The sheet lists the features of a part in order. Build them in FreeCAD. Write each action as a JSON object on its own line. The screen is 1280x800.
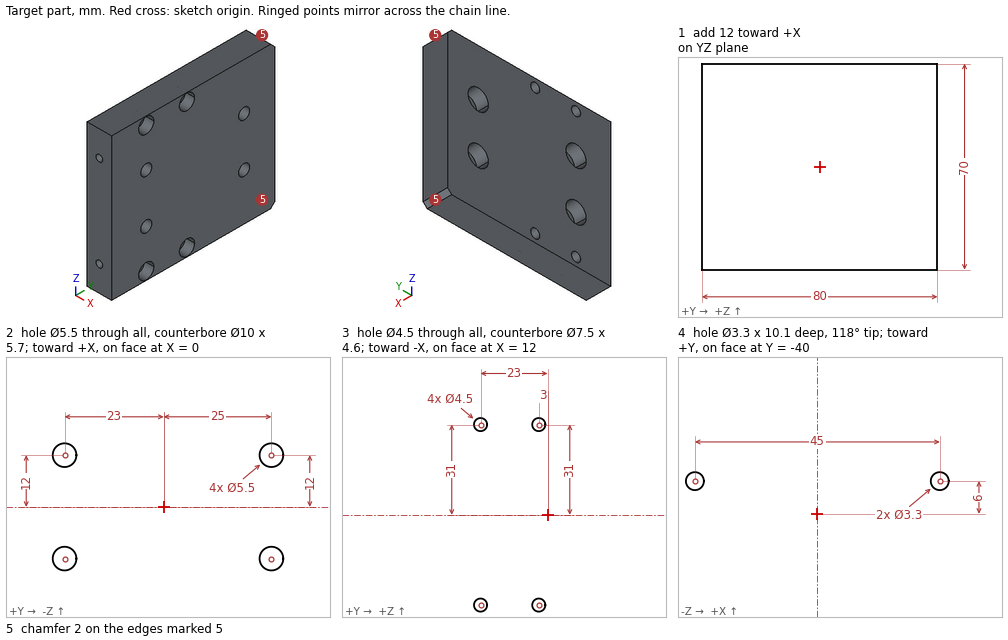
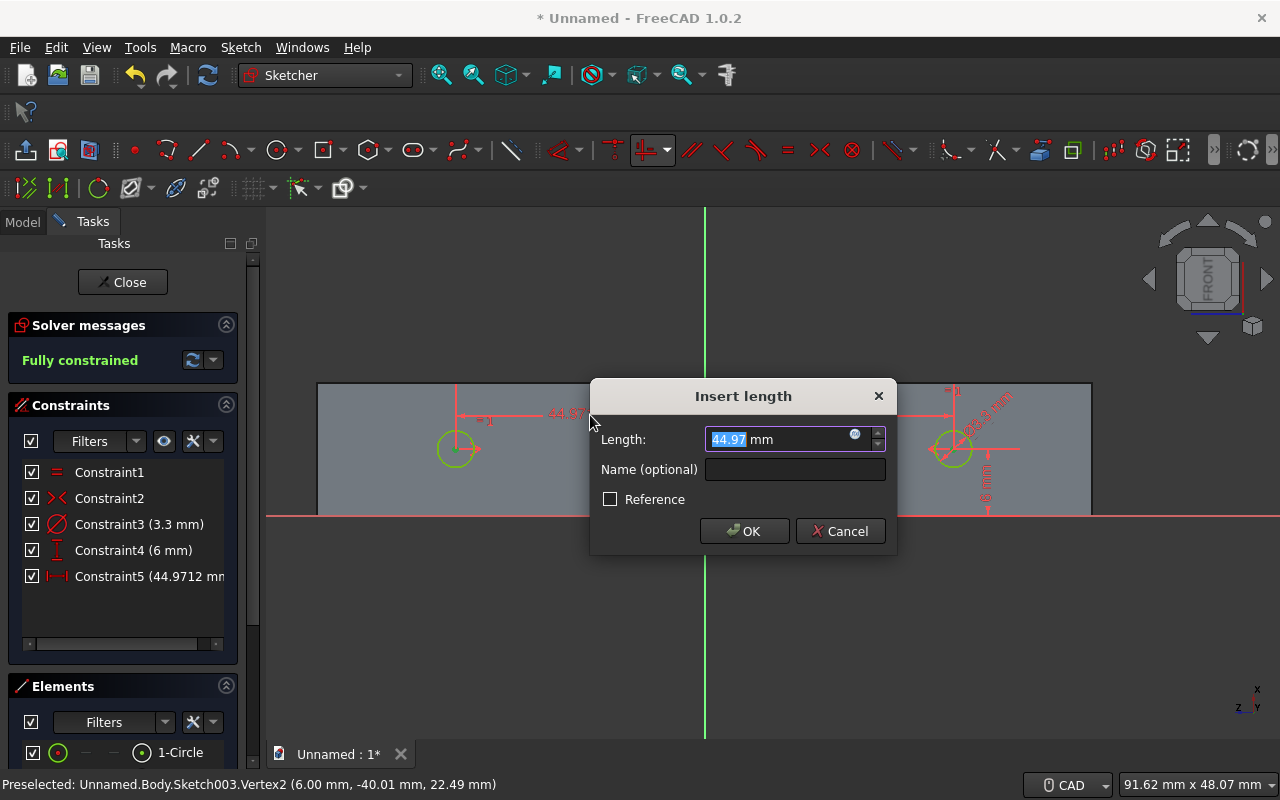
{"action": "type", "text": "45"}
{"action": "key", "text": "Return"}
{"action": "key", "text": "Escape"}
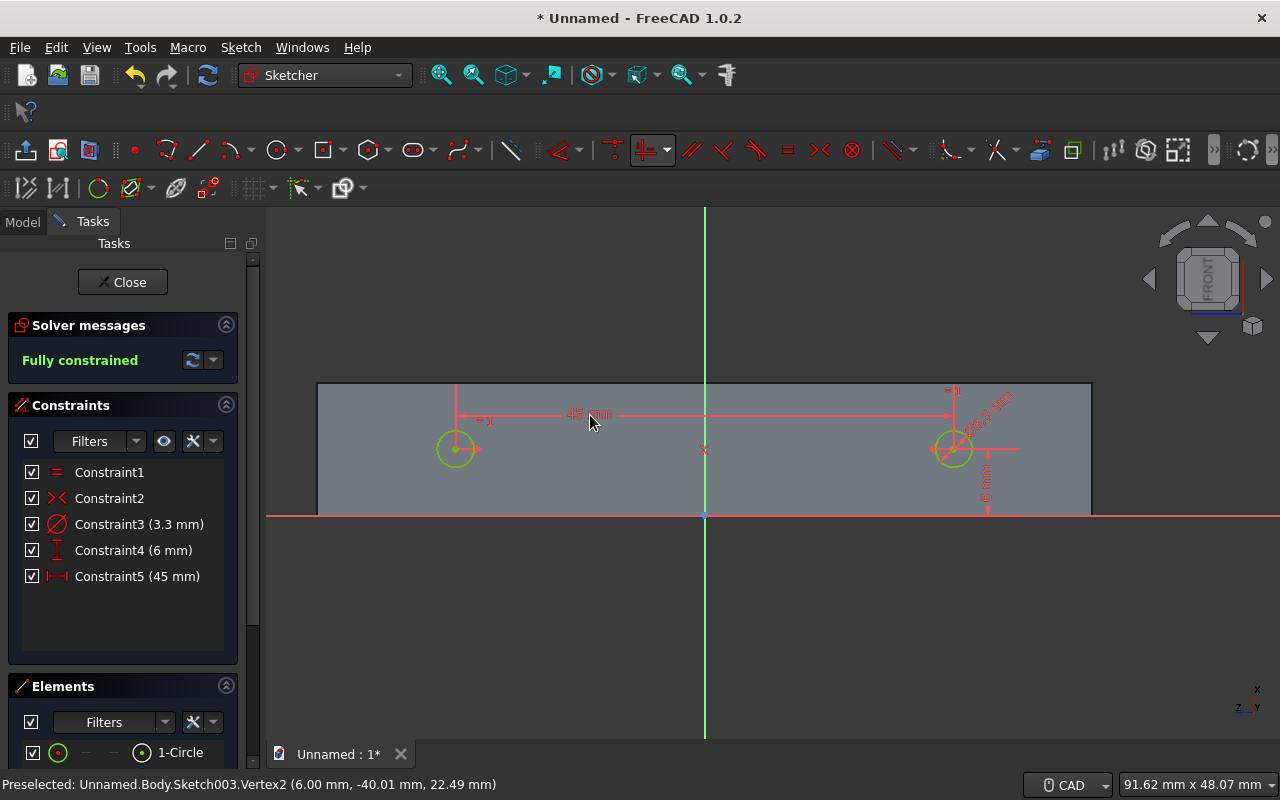
{"action": "left_click", "coordinate": [123, 282]}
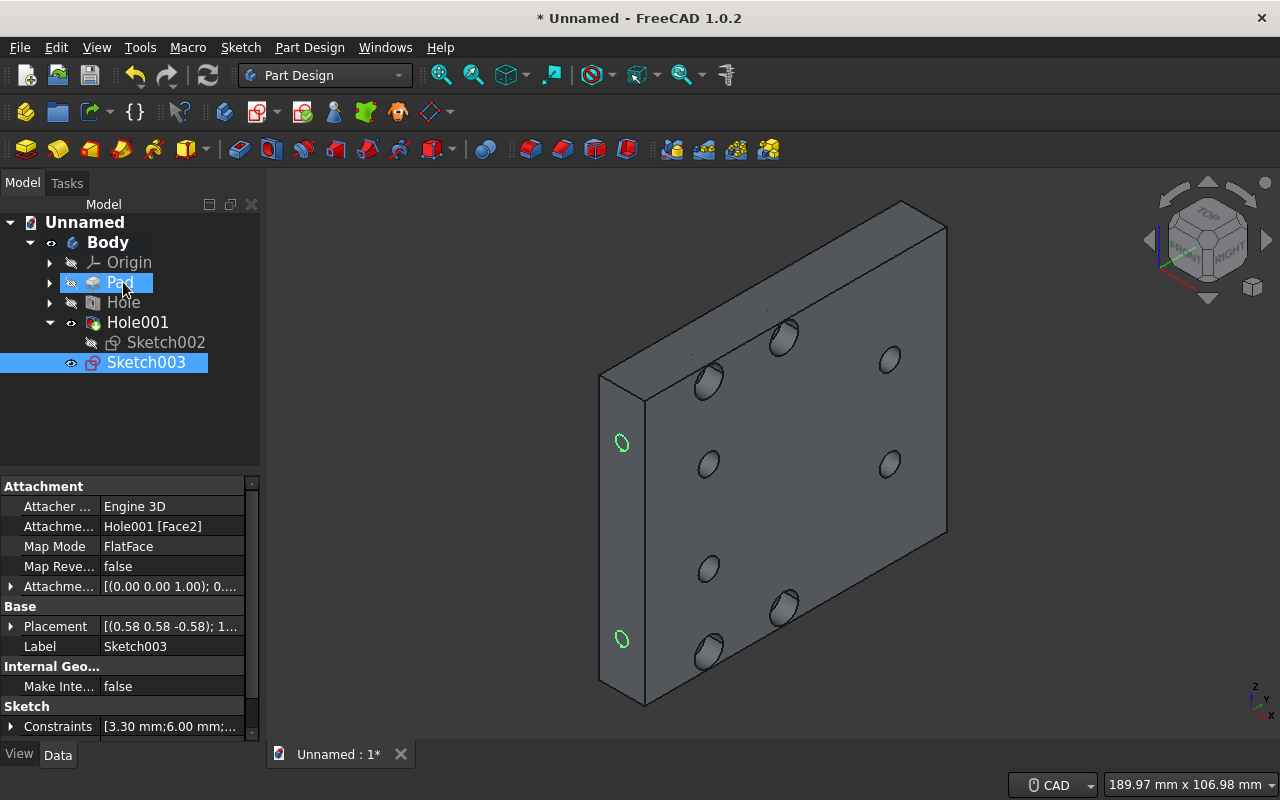
{"action": "left_click", "coordinate": [272, 150]}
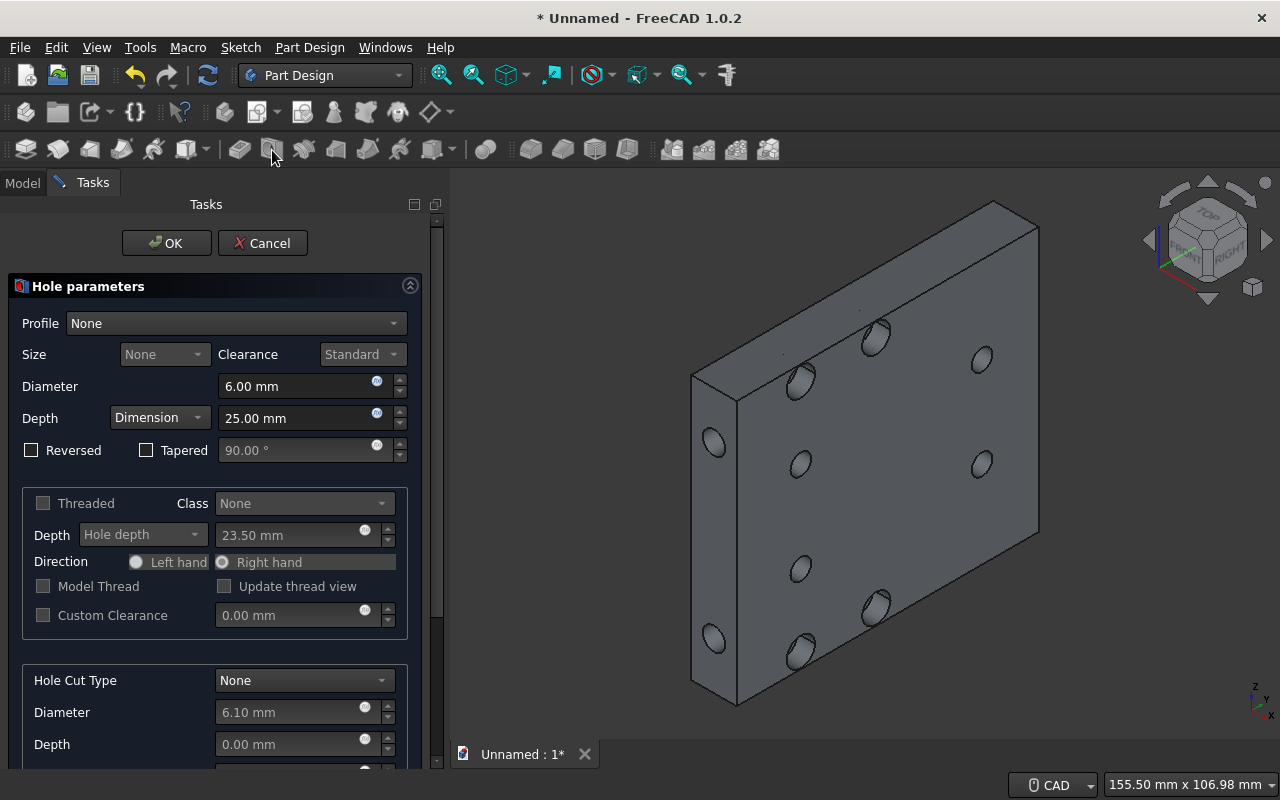
{"action": "triple_click", "coordinate": [305, 386]}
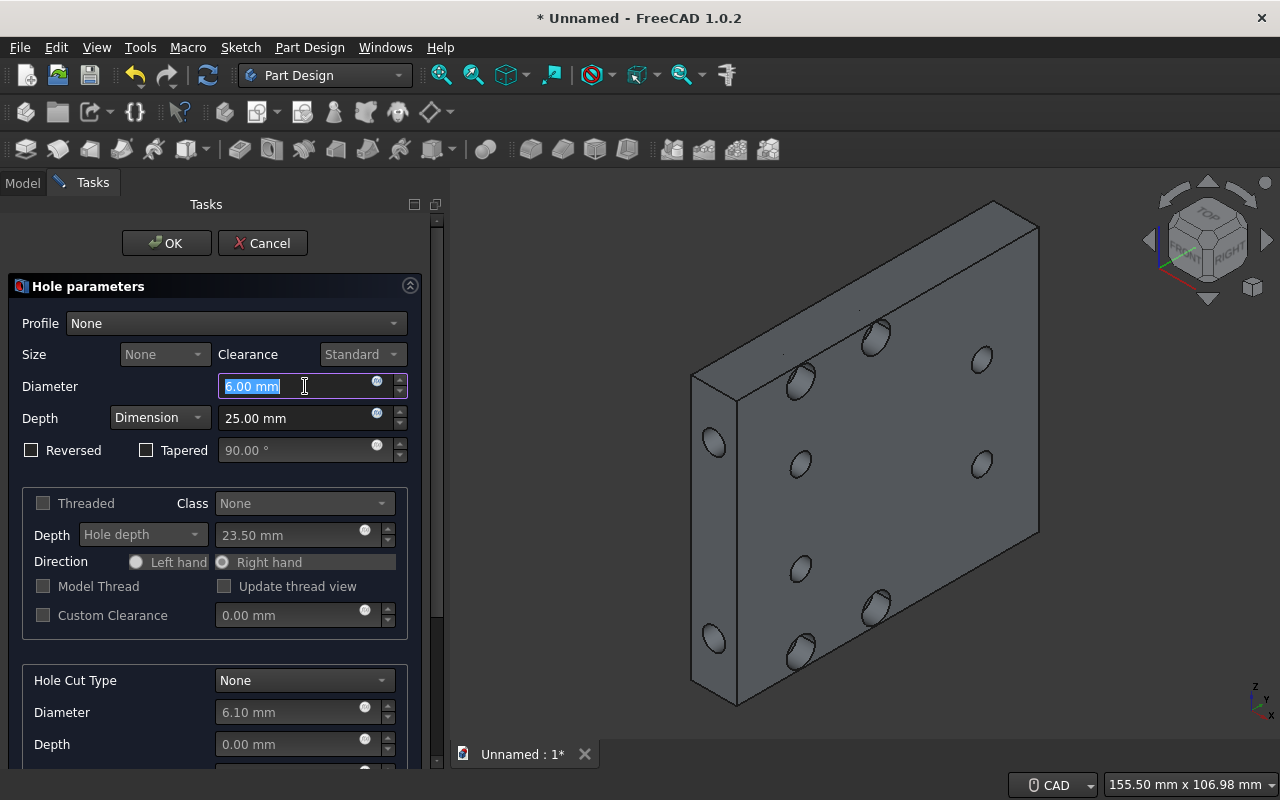
{"action": "type", "text": "3.3"}
{"action": "key", "text": "Tab"}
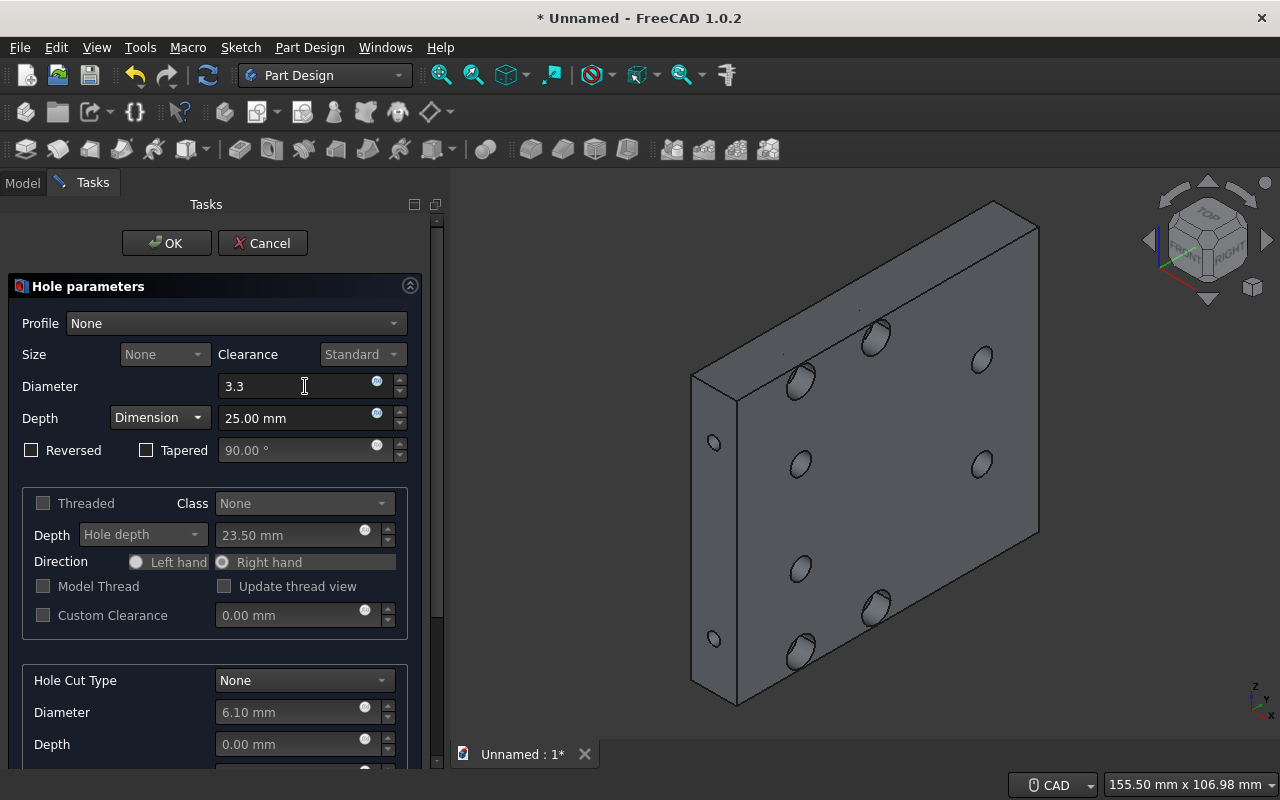
{"action": "triple_click", "coordinate": [305, 418]}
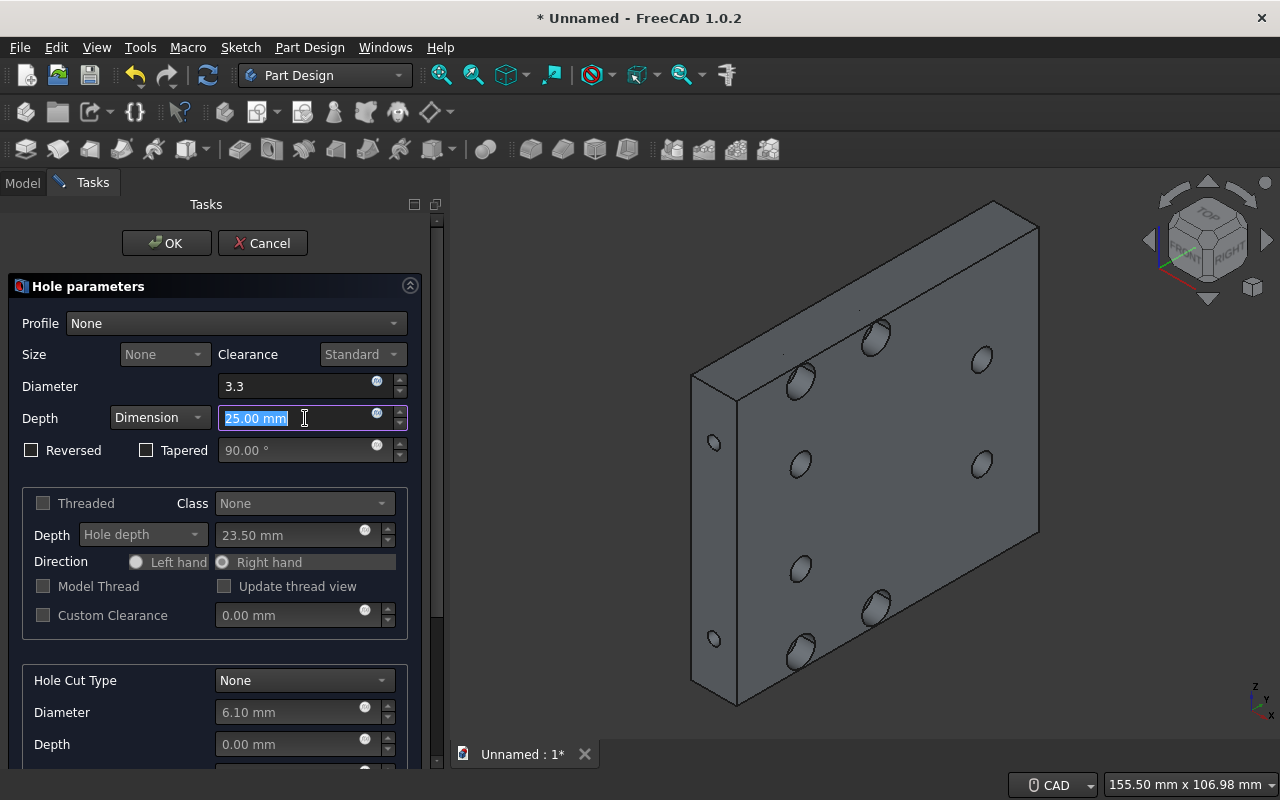
{"action": "type", "text": "10.1"}
{"action": "key", "text": "Tab"}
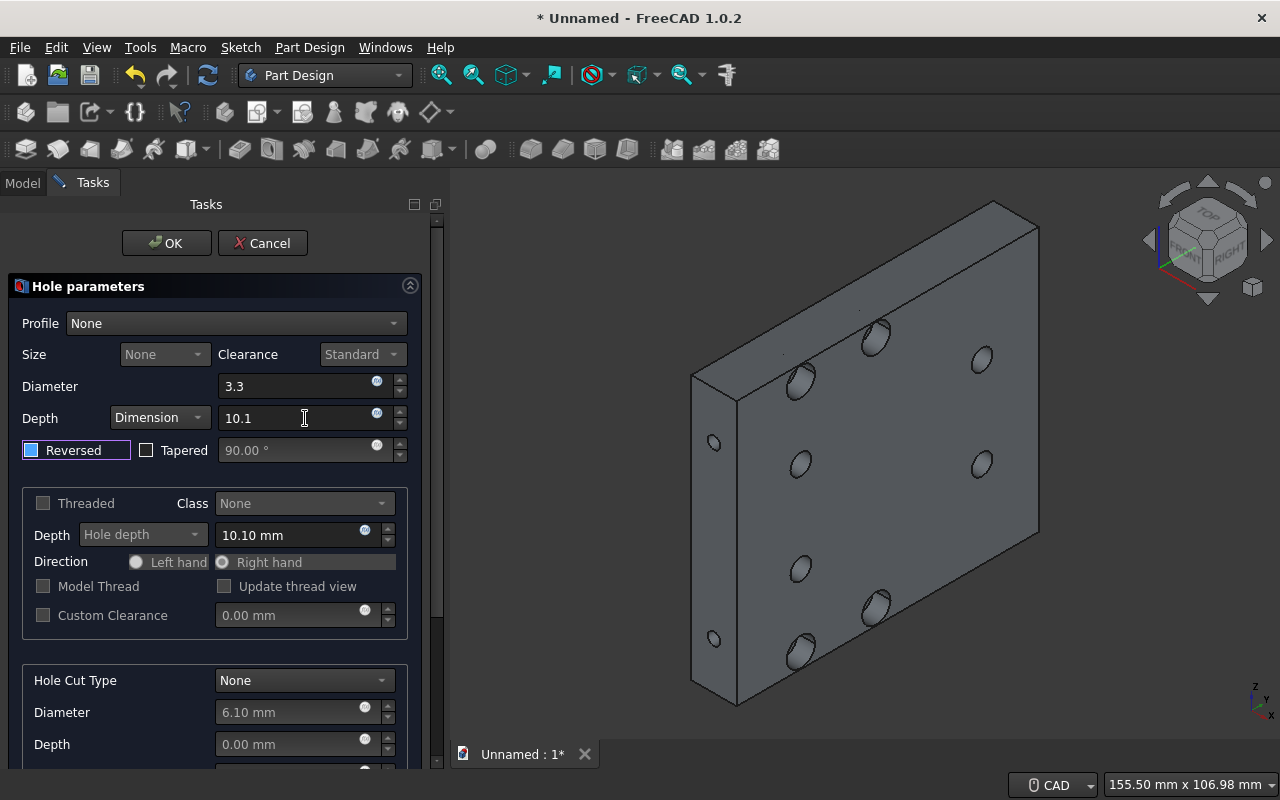
{"action": "left_click", "coordinate": [167, 243]}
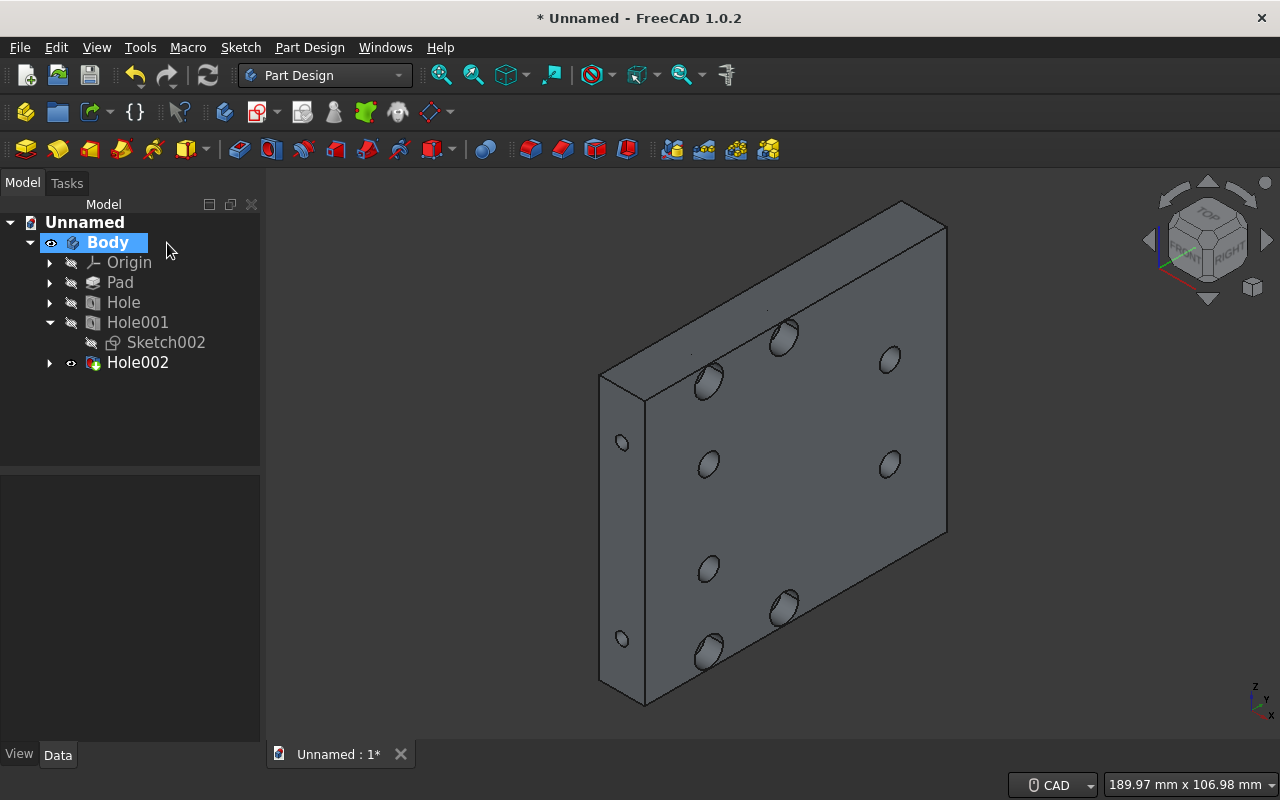
{"action": "key", "text": "2"}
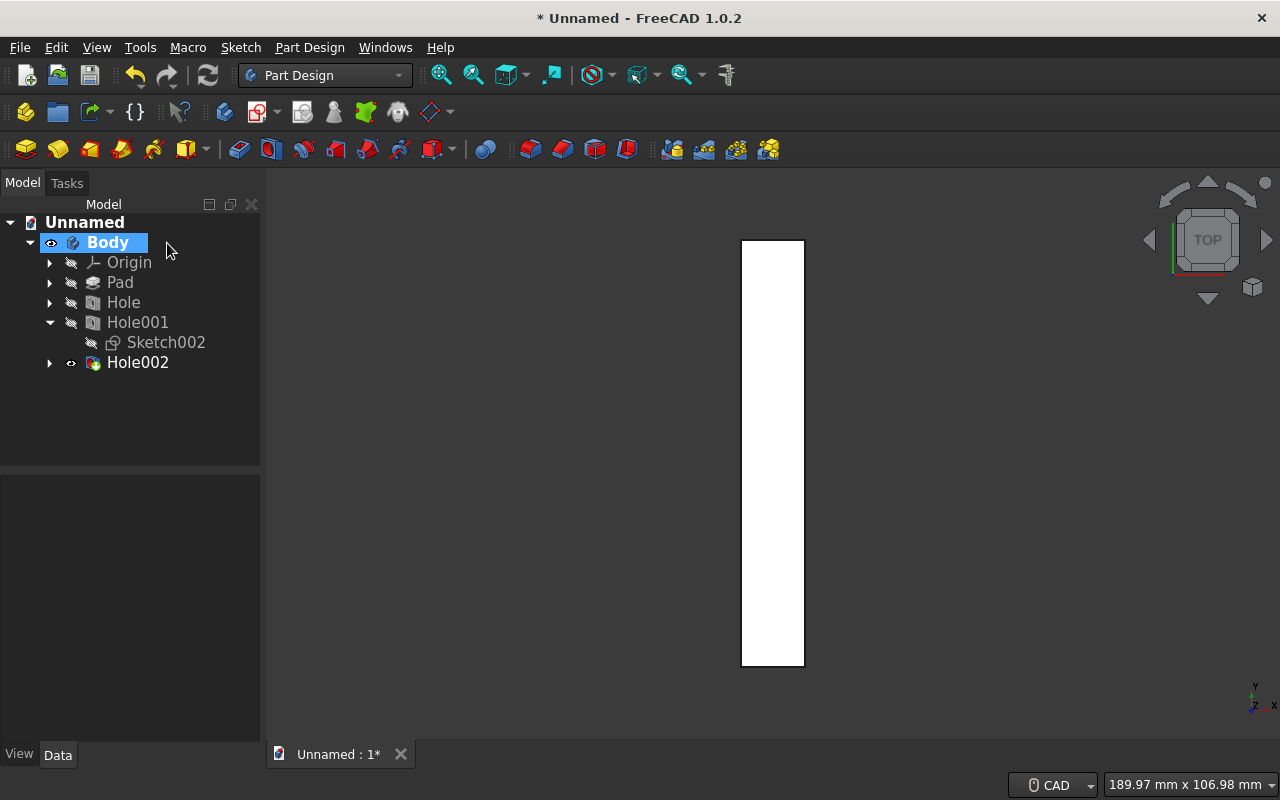
{"action": "left_click", "coordinate": [773, 239]}